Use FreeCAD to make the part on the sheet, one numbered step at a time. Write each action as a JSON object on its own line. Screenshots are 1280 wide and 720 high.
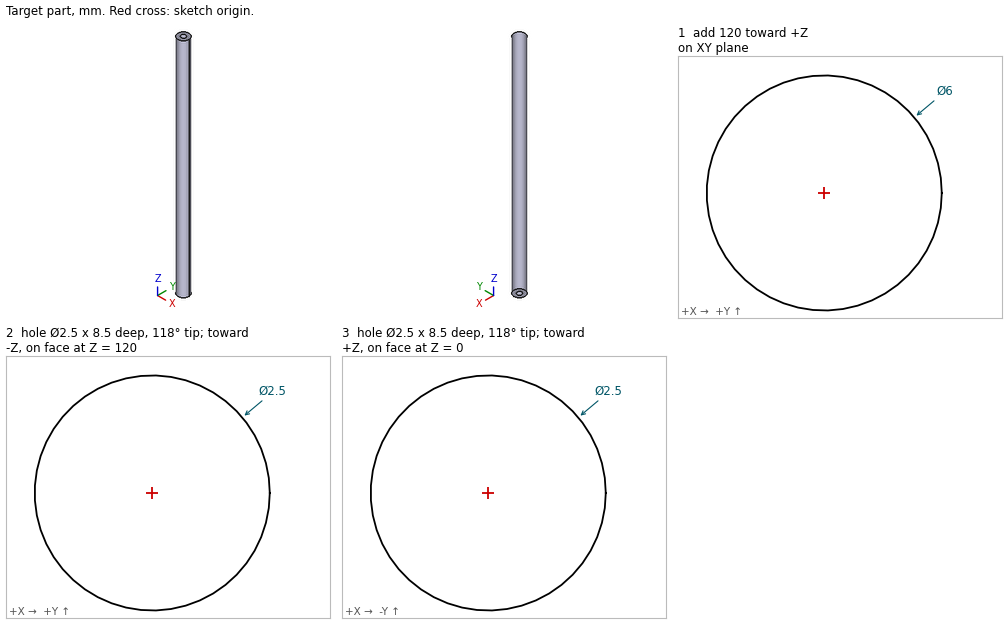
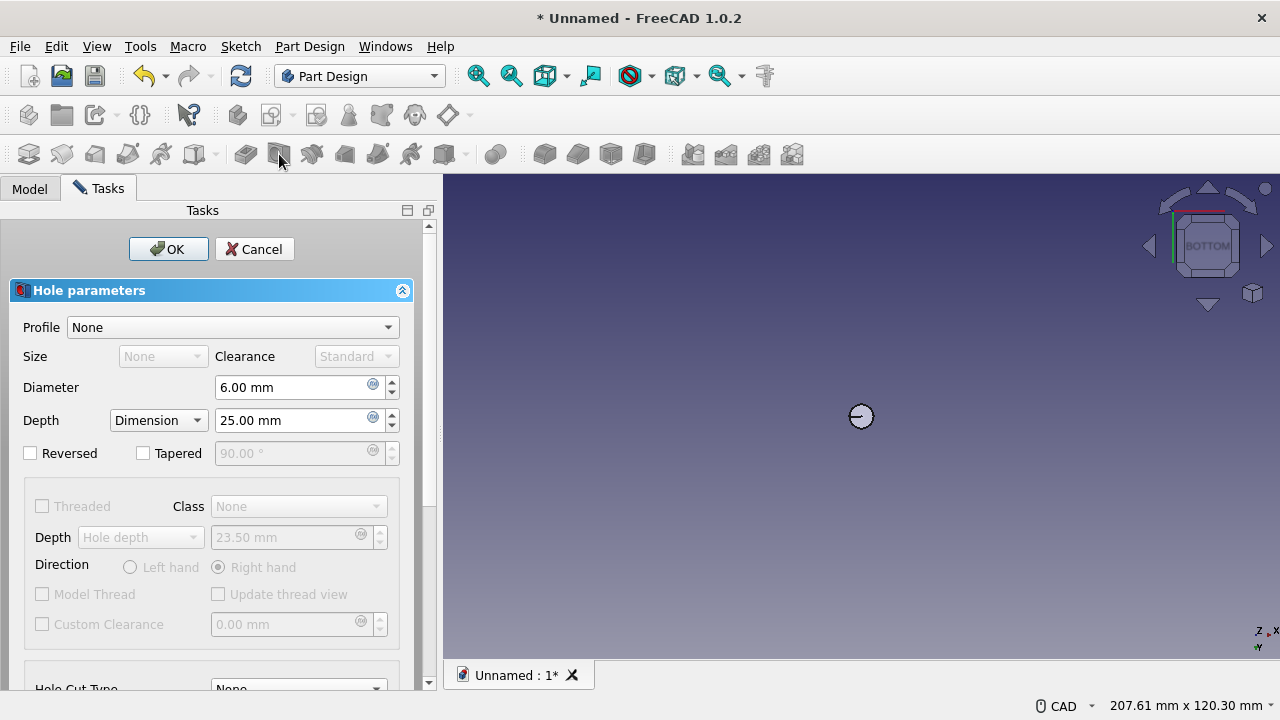
{"action": "triple_click", "coordinate": [300, 388]}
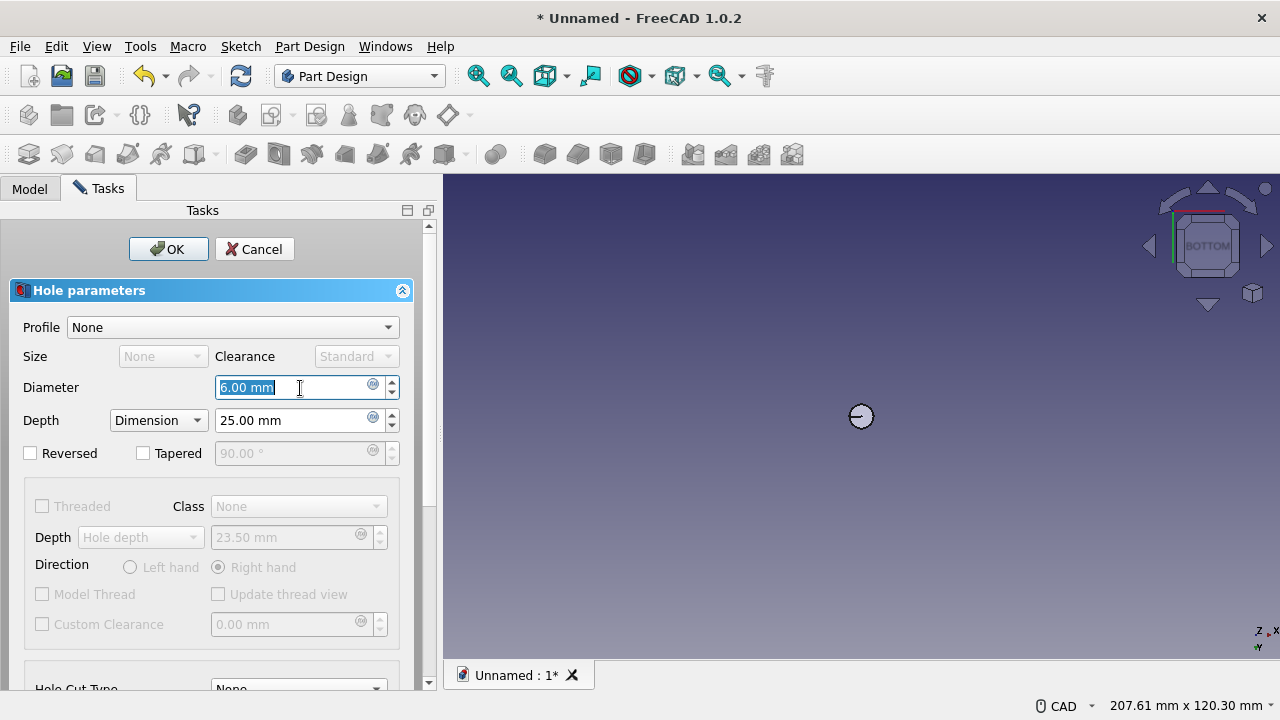
{"action": "type", "text": "2.5"}
{"action": "key", "text": "Tab"}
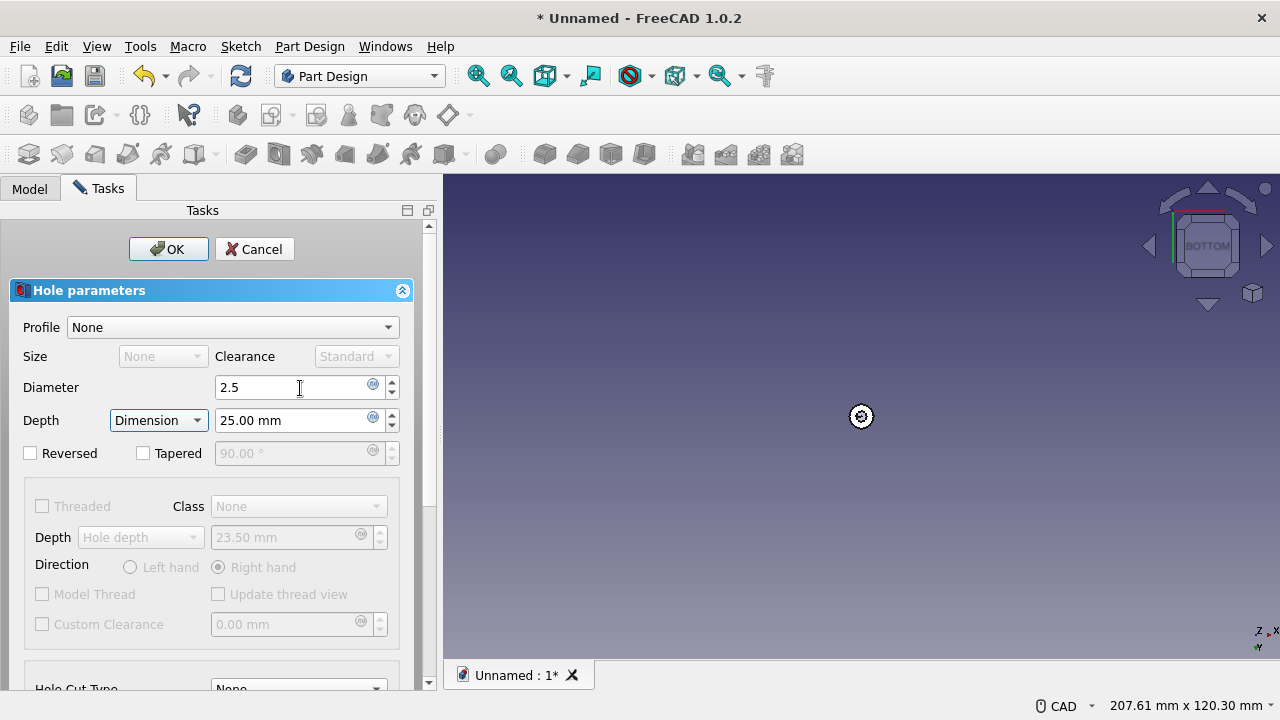
{"action": "triple_click", "coordinate": [300, 420]}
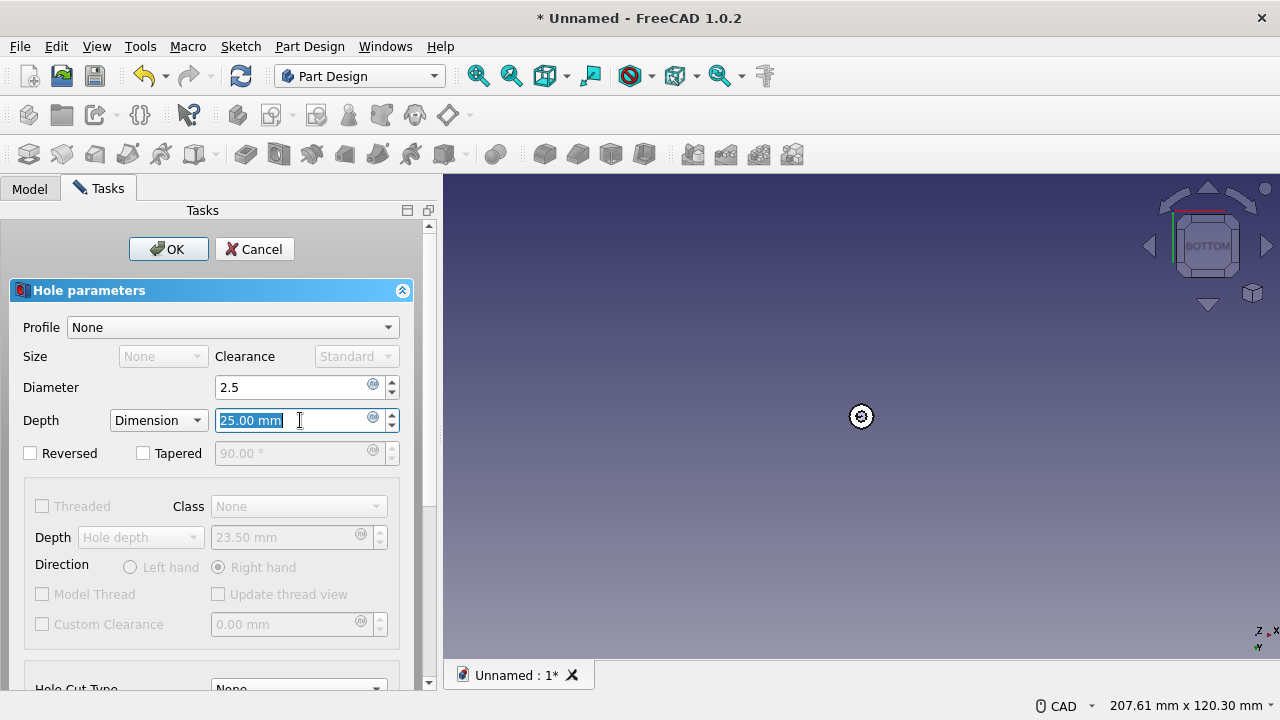
{"action": "type", "text": "8.5"}
{"action": "key", "text": "Tab"}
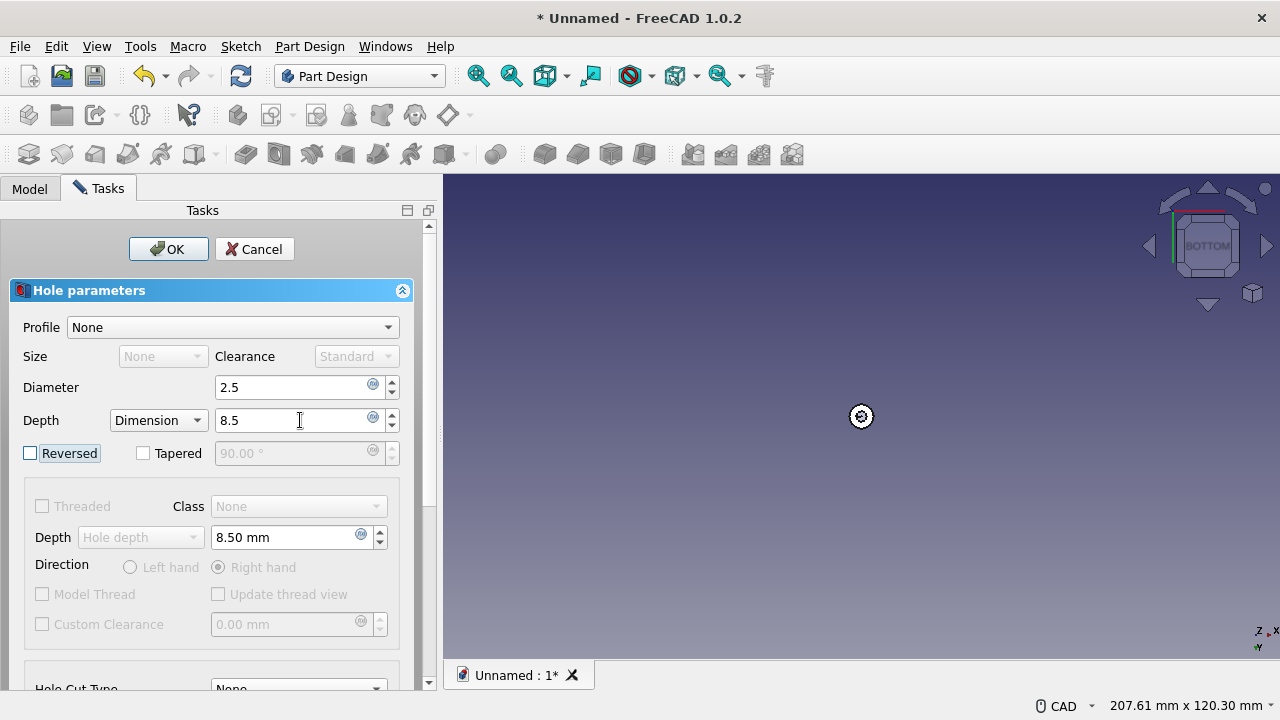
{"action": "left_click", "coordinate": [169, 249]}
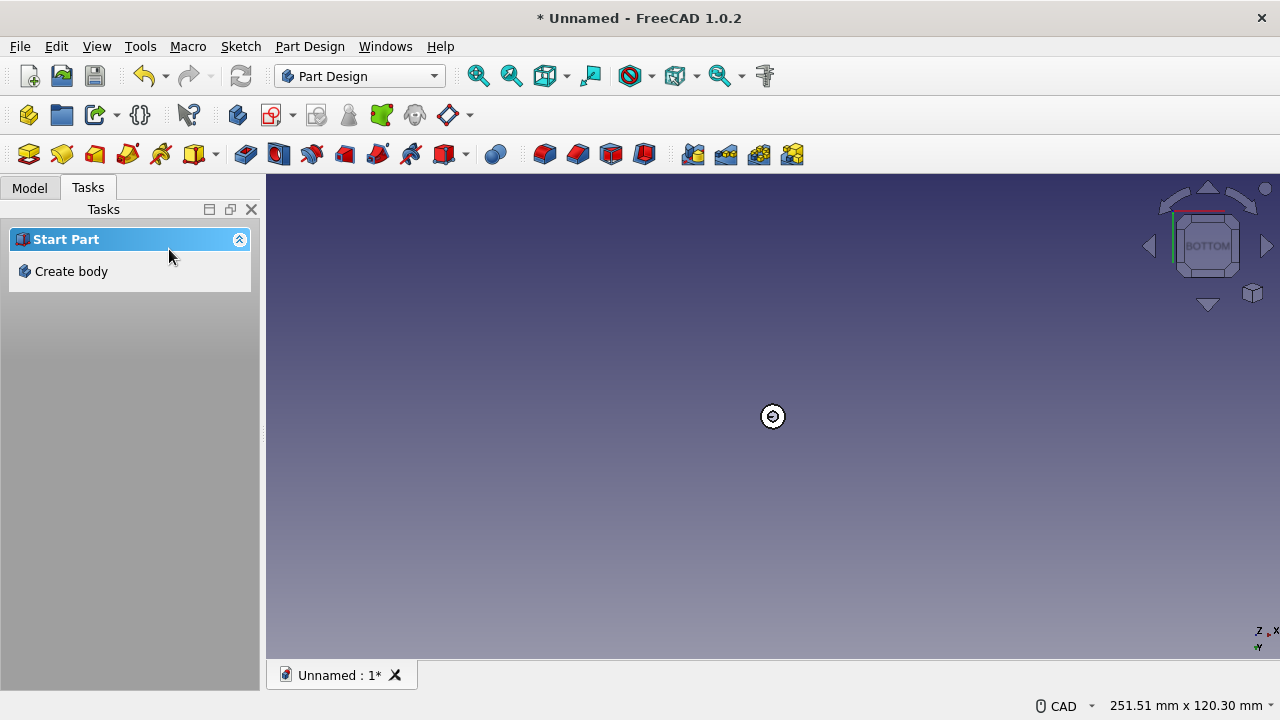
{"action": "key", "text": "0"}